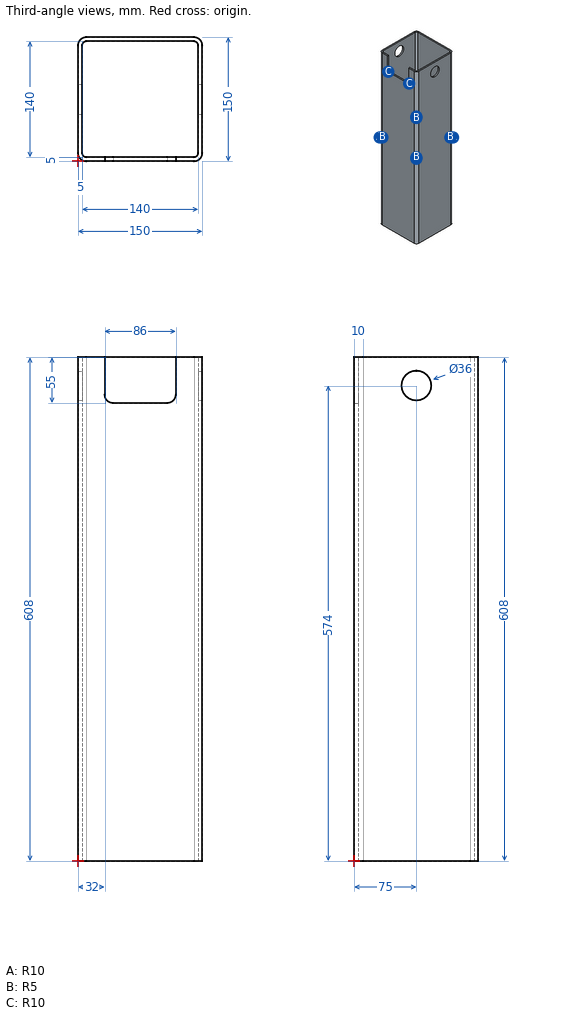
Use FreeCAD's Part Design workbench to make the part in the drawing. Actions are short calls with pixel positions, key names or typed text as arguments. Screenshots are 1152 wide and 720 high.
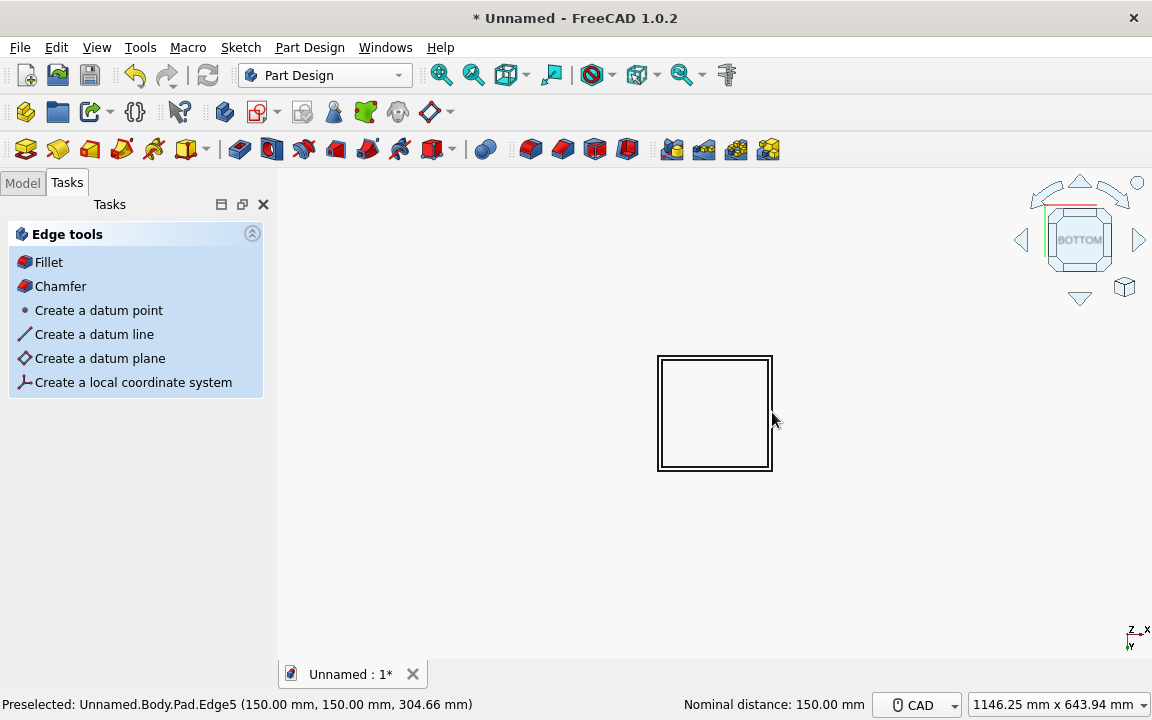
key(v)
key(f)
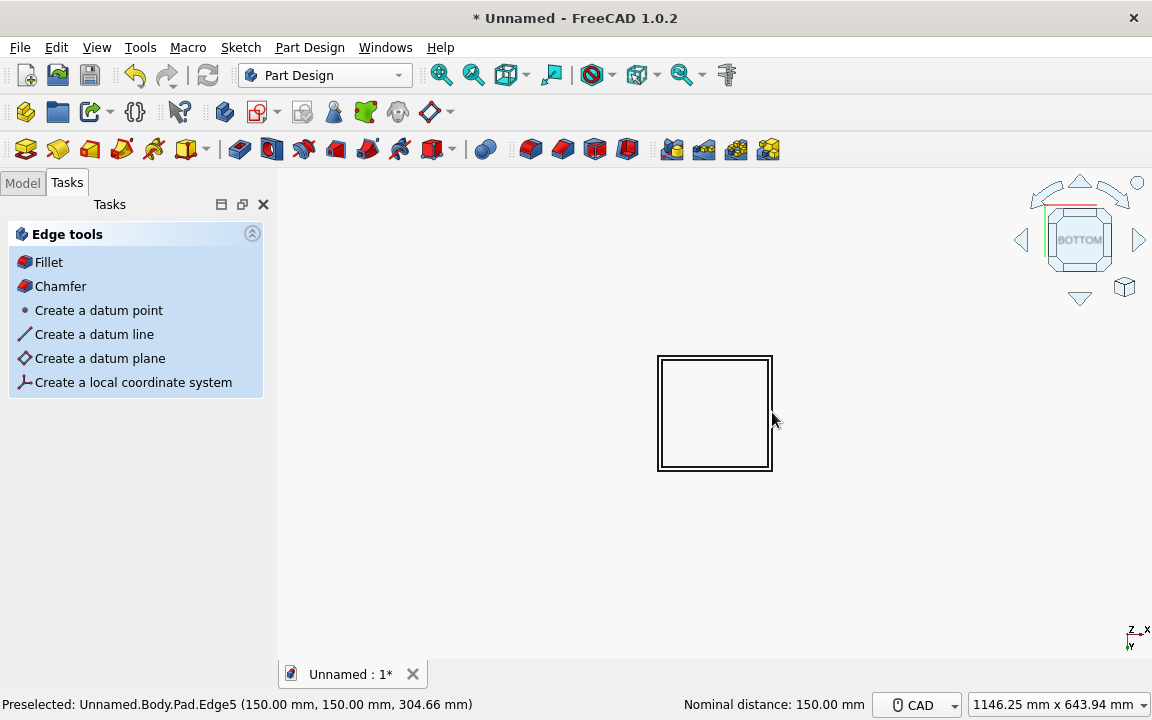
key(4)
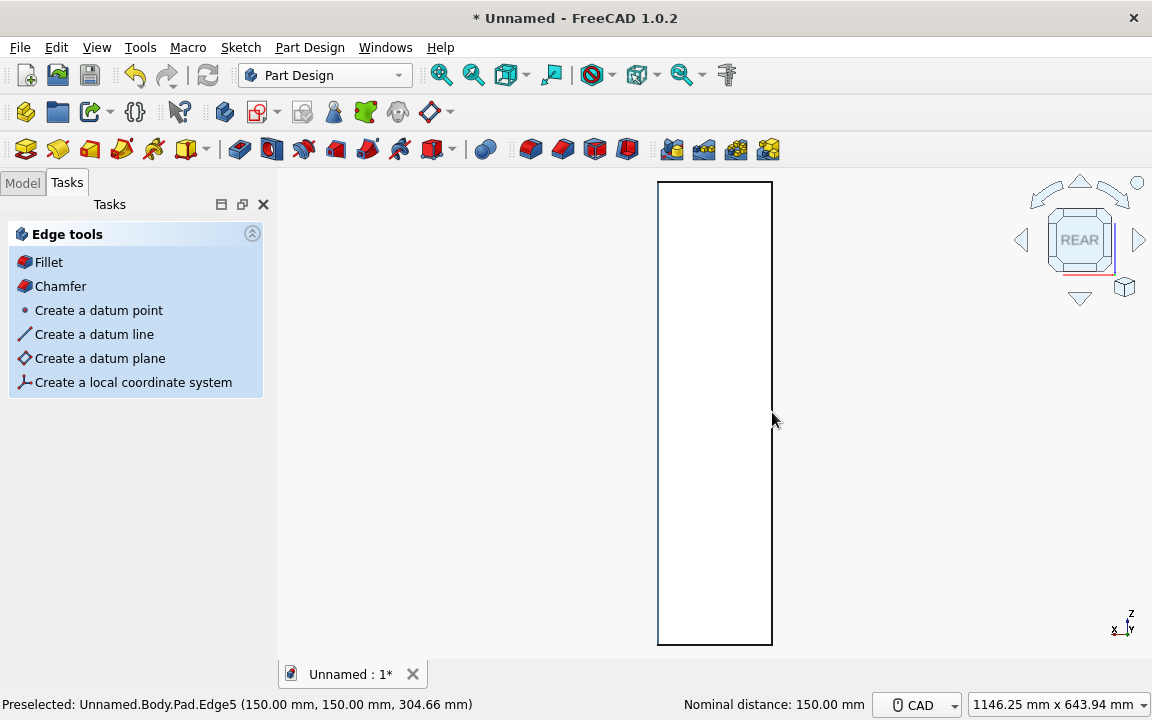
click(772, 413, ctrl)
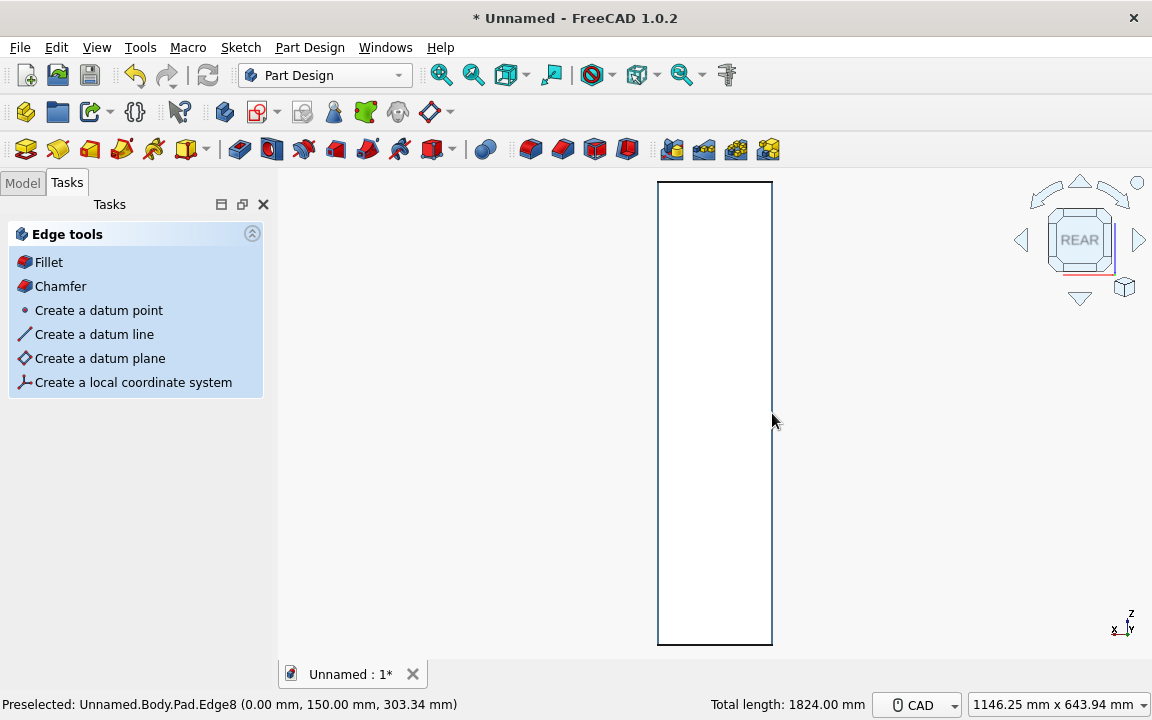
key(6)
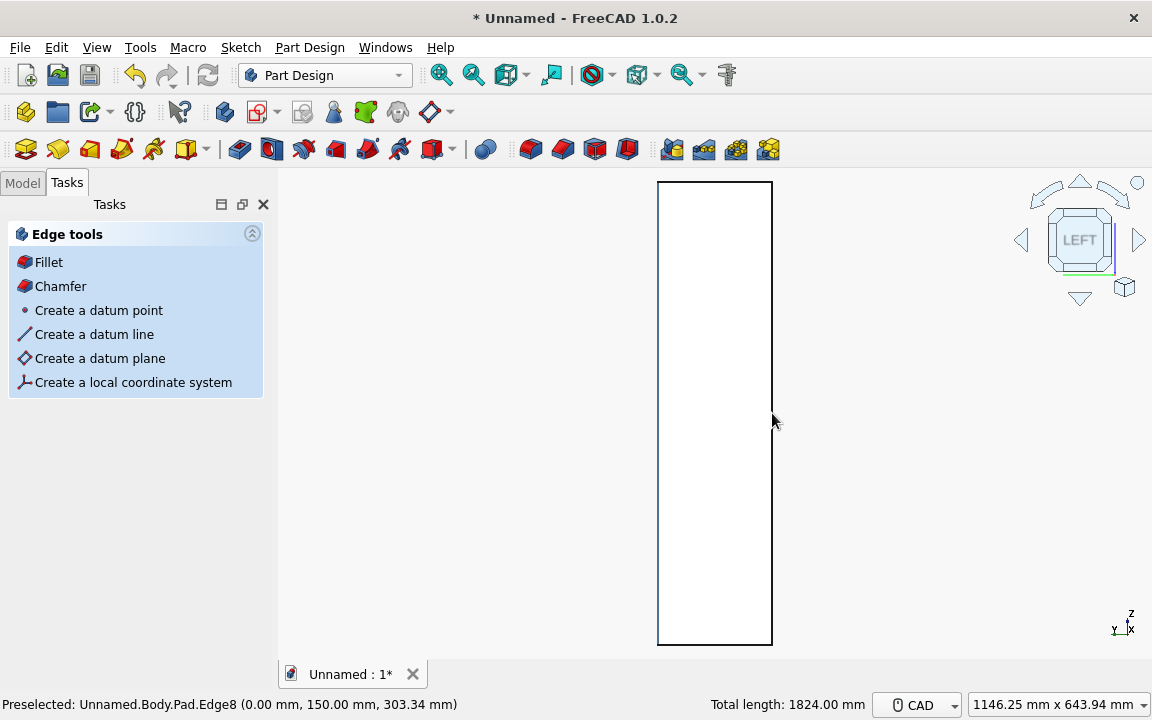
key(v)
key(3)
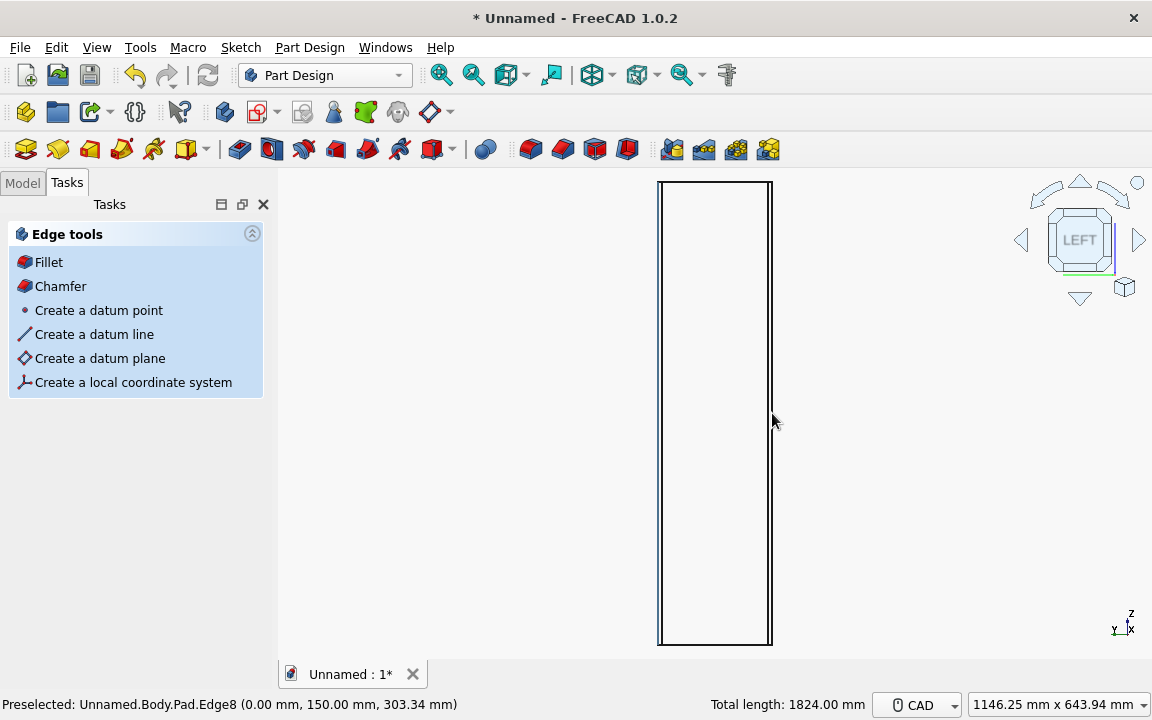
key(0)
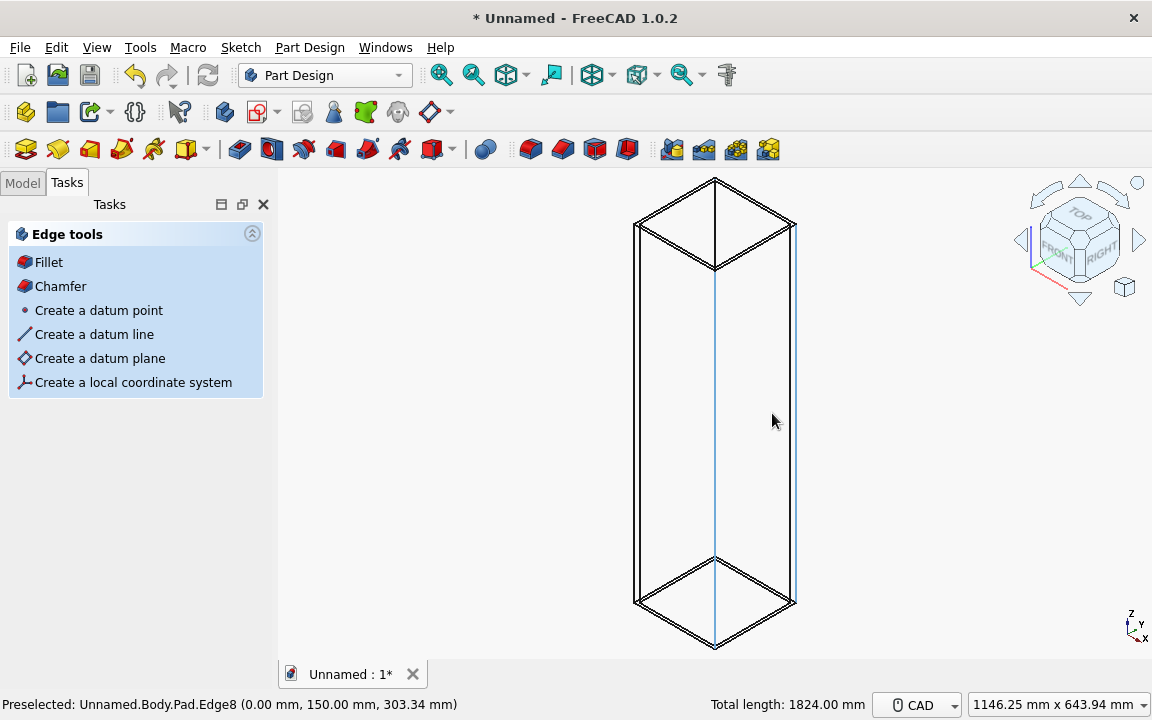
scroll(634, 412, up, 6)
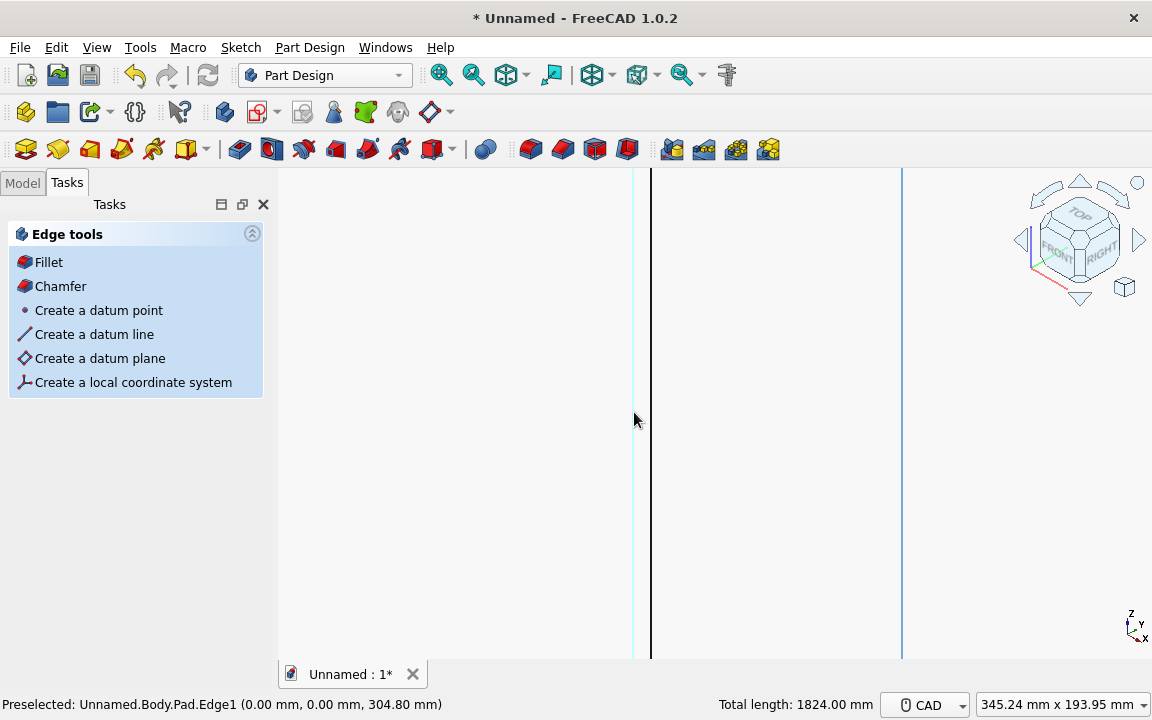
click(633, 415, ctrl)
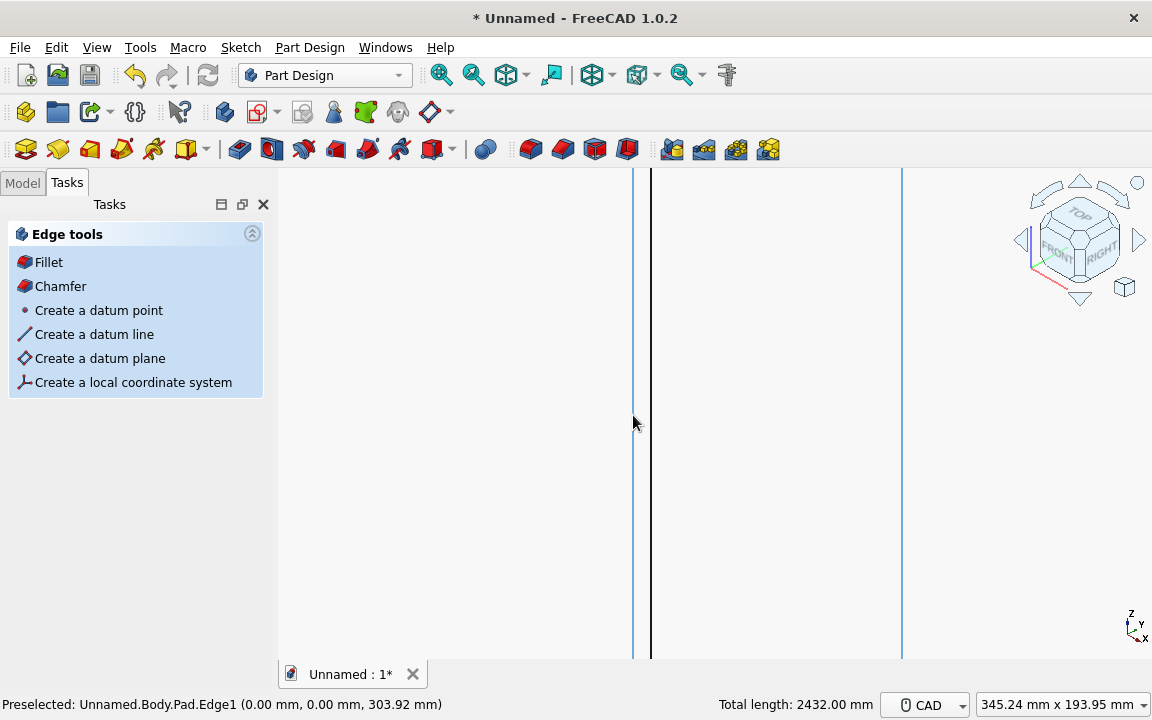
key(v)
key(1)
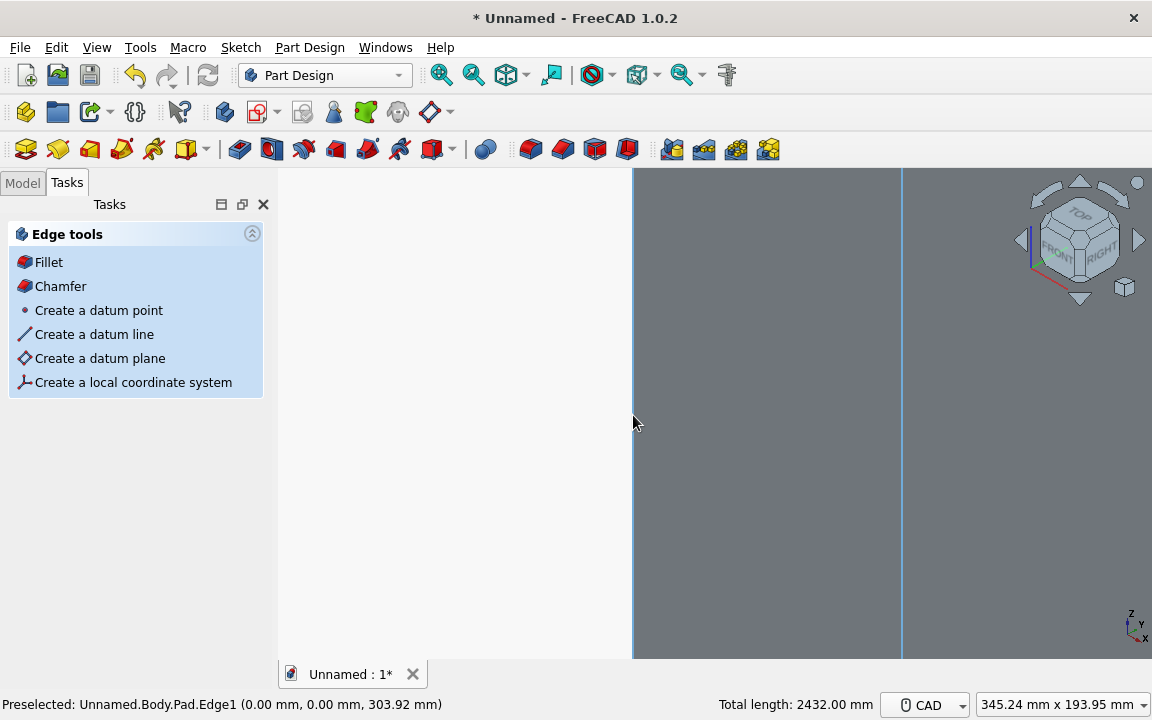
click(532, 150)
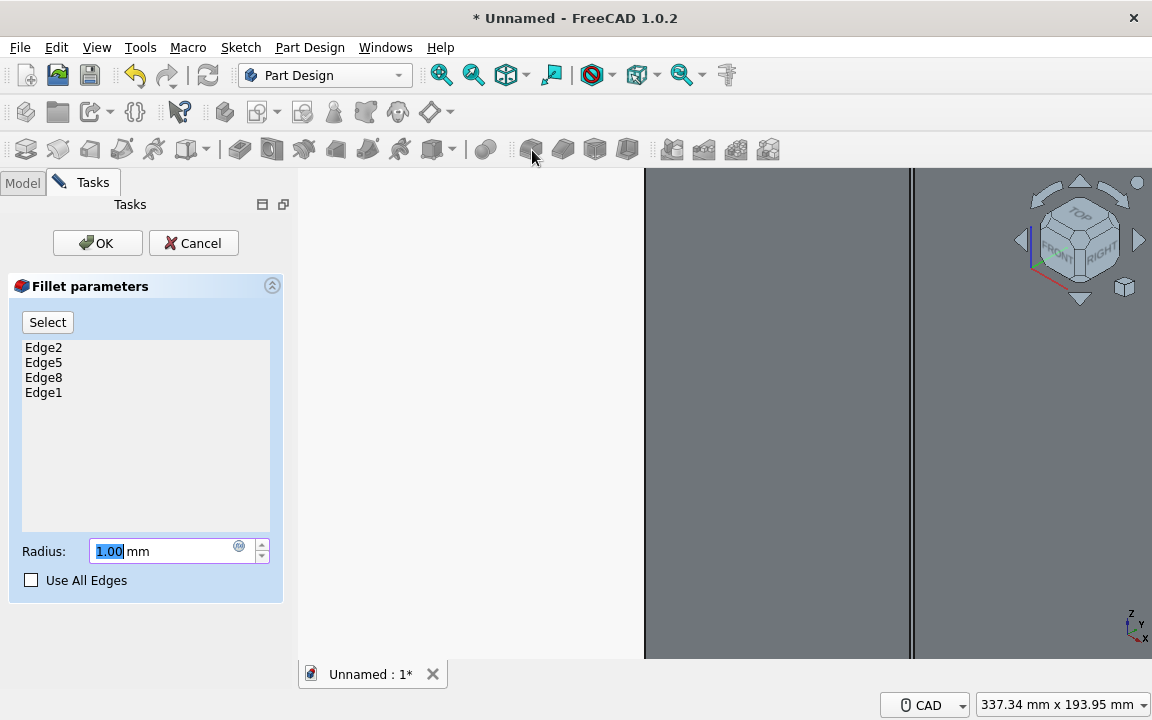
text(10)
key(Tab)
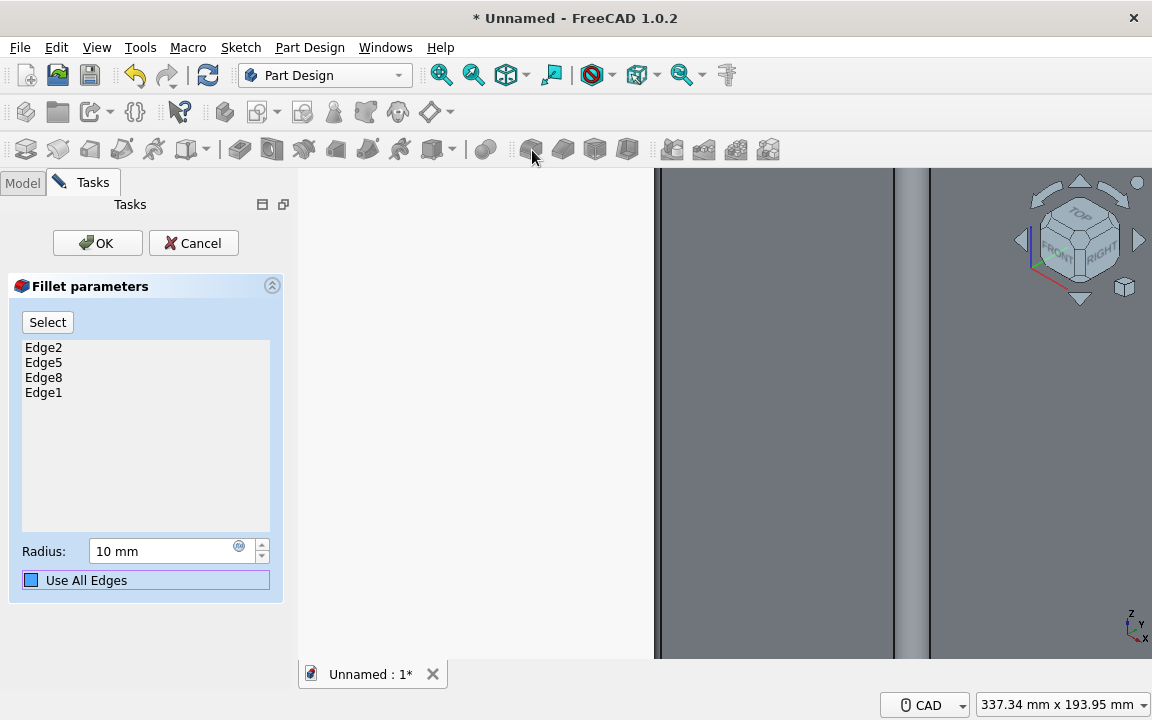
click(98, 243)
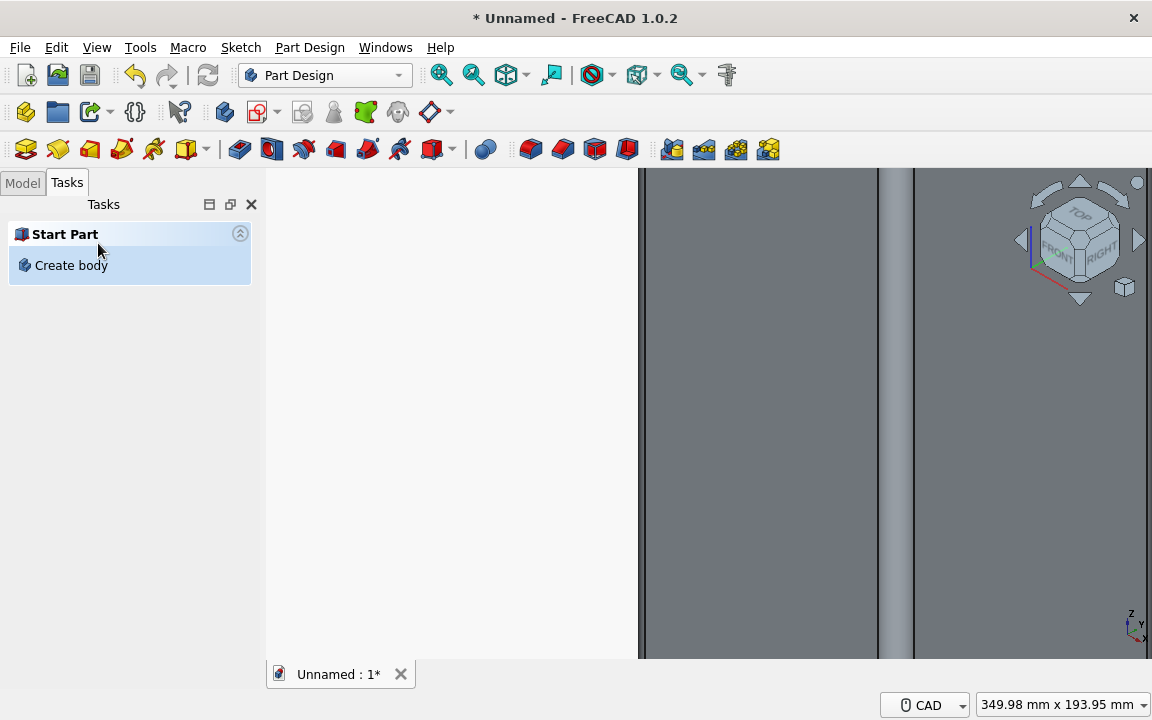
key(v)
key(f)